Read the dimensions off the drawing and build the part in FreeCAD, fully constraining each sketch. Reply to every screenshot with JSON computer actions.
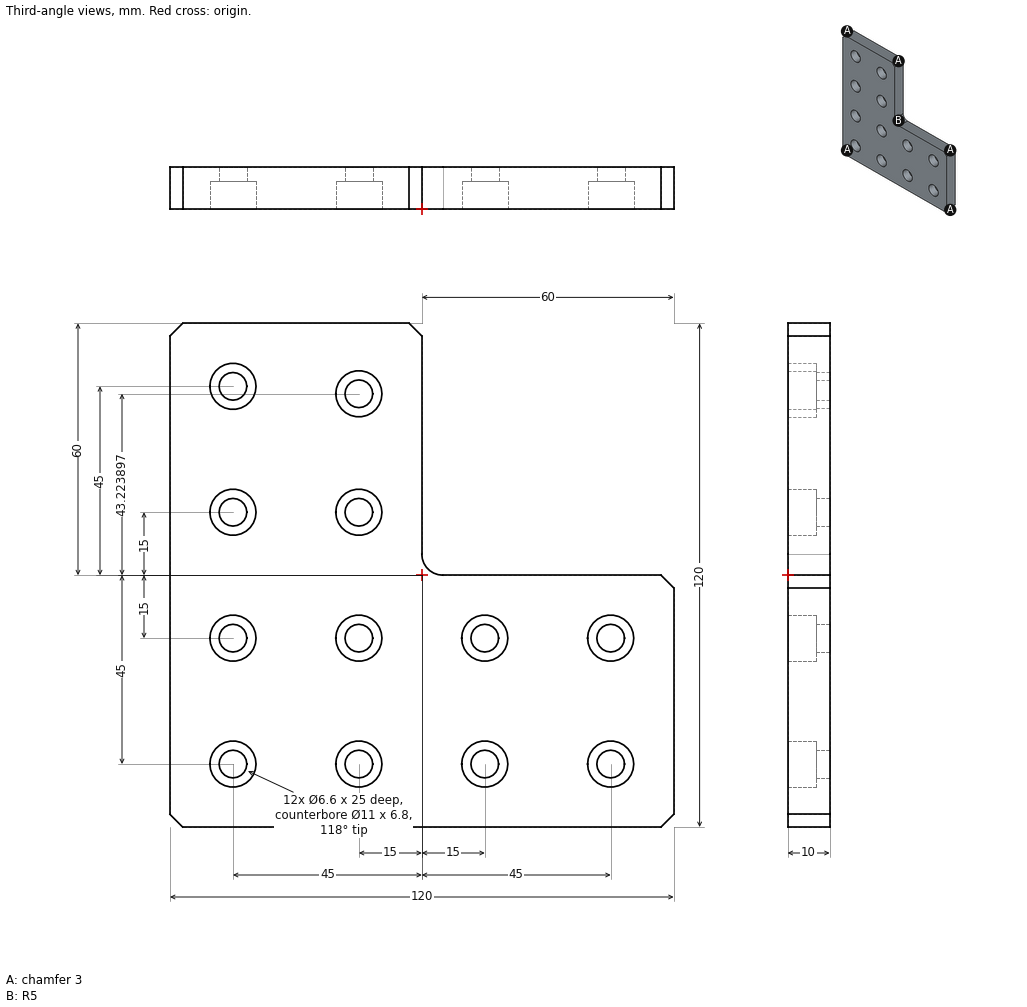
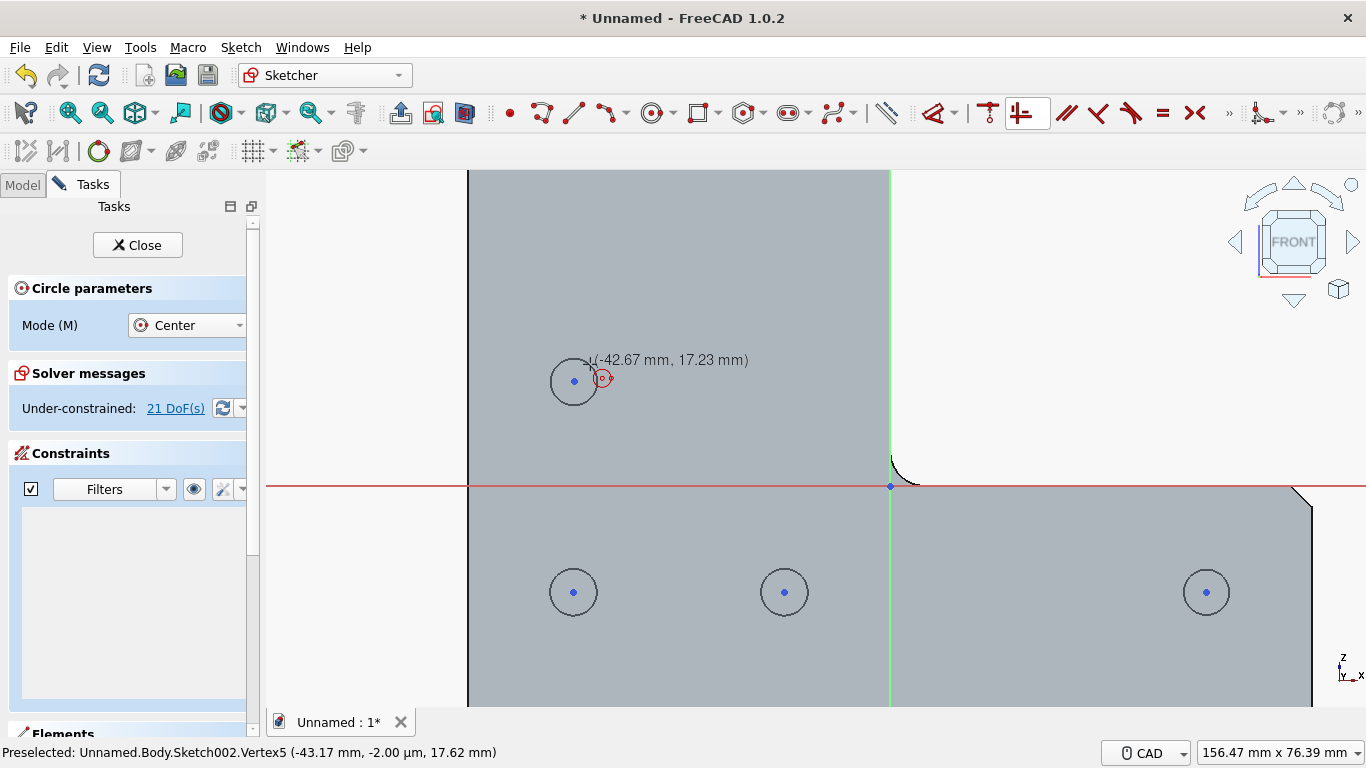
{"action": "scroll", "coordinate": [574, 381], "scroll_direction": "down", "scroll_amount": 3}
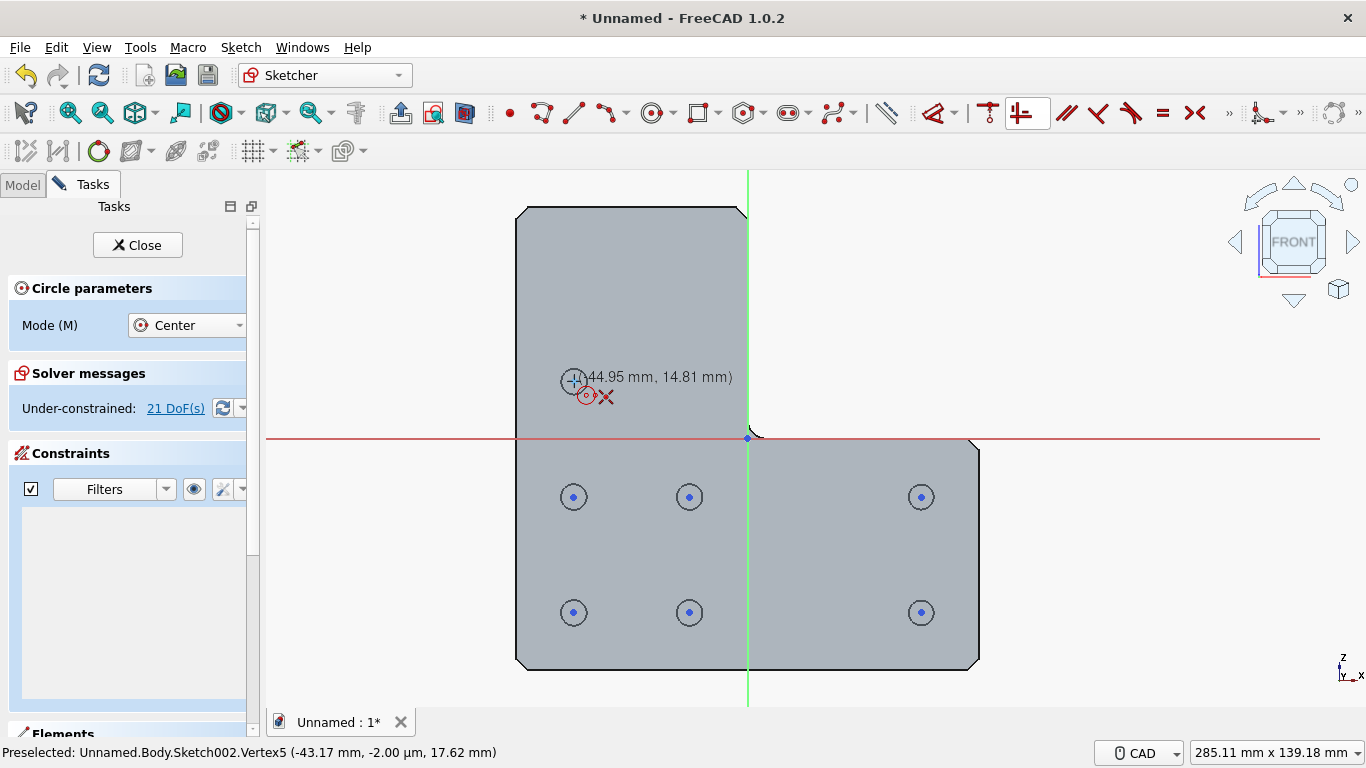
{"action": "scroll", "coordinate": [574, 265], "scroll_direction": "up", "scroll_amount": 3}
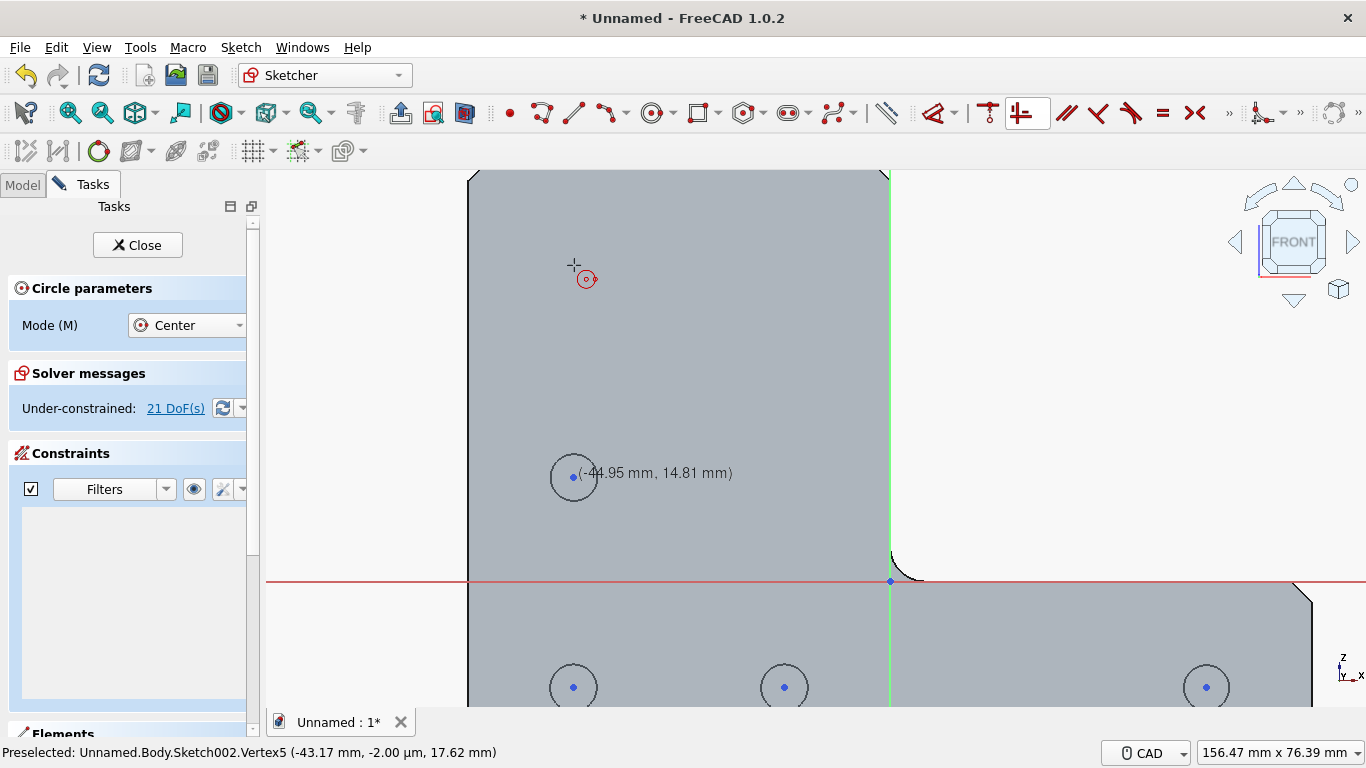
{"action": "left_click", "coordinate": [574, 265]}
{"action": "left_click", "coordinate": [590, 249]}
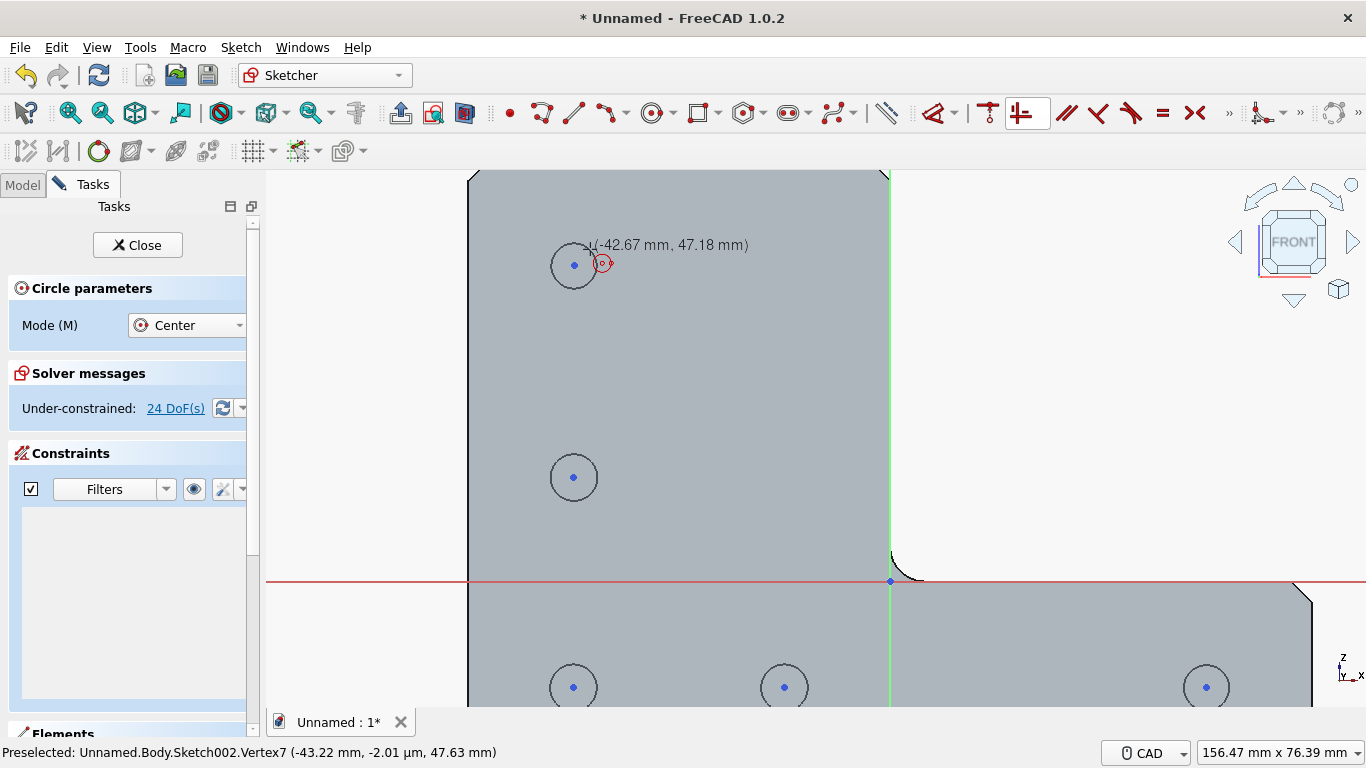
{"action": "left_click", "coordinate": [785, 278]}
{"action": "left_click", "coordinate": [801, 261]}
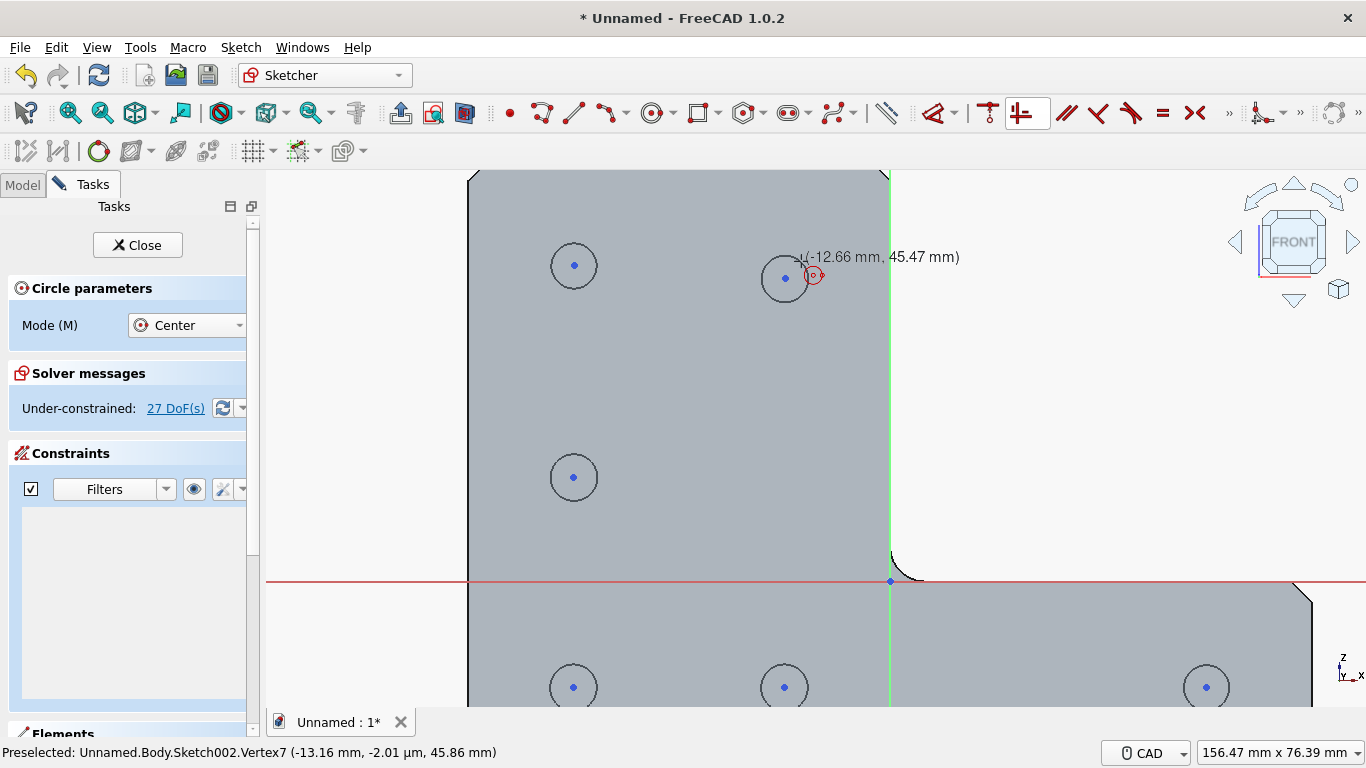
{"action": "left_click", "coordinate": [785, 476]}
{"action": "left_click", "coordinate": [801, 460]}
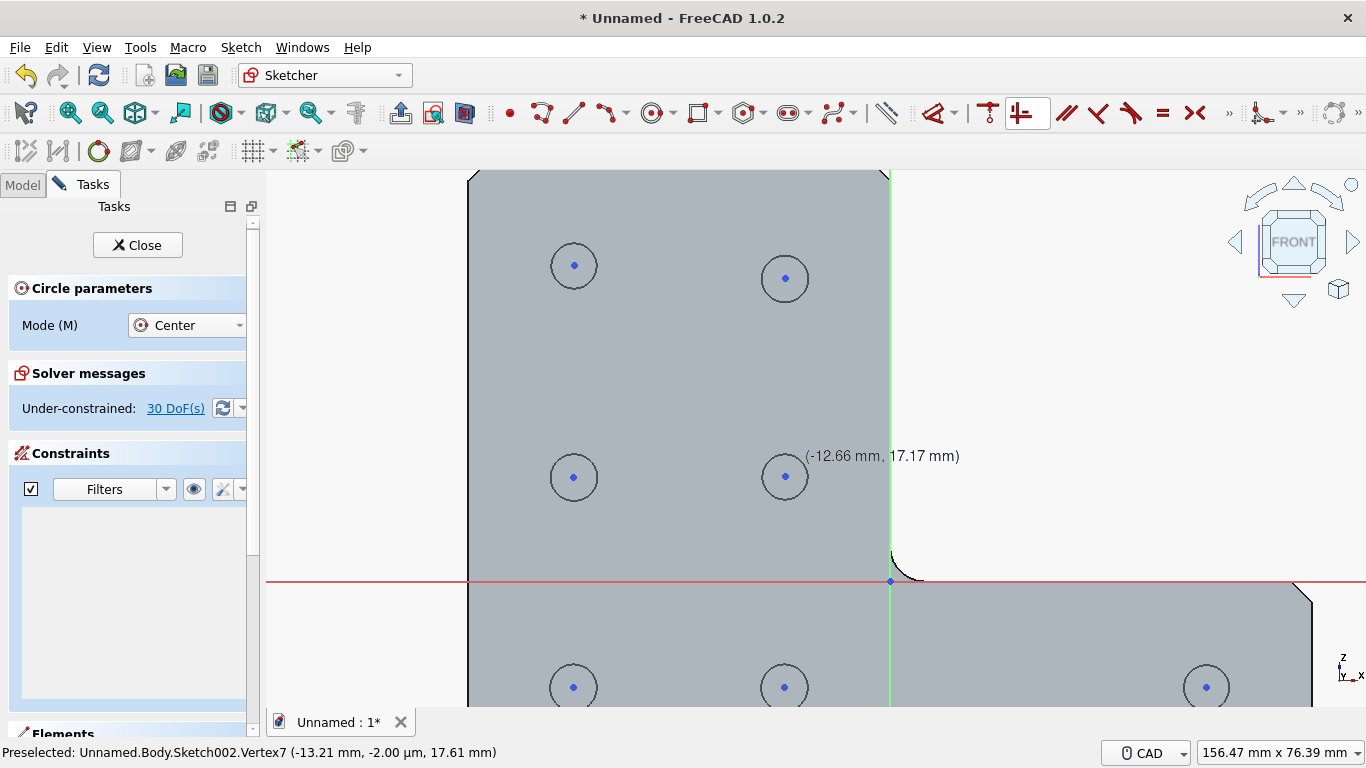
{"action": "scroll", "coordinate": [574, 264], "scroll_direction": "down", "scroll_amount": 3}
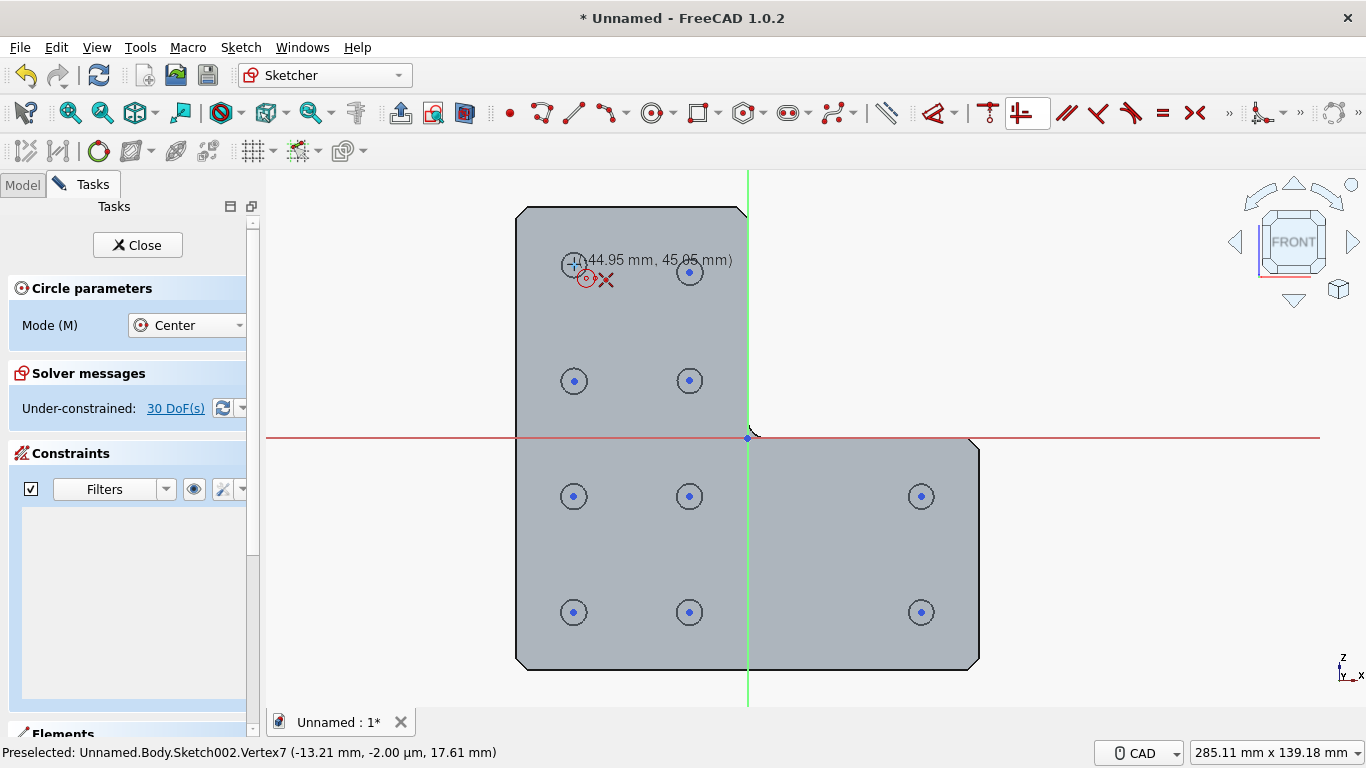
{"action": "scroll", "coordinate": [805, 612], "scroll_direction": "up", "scroll_amount": 3}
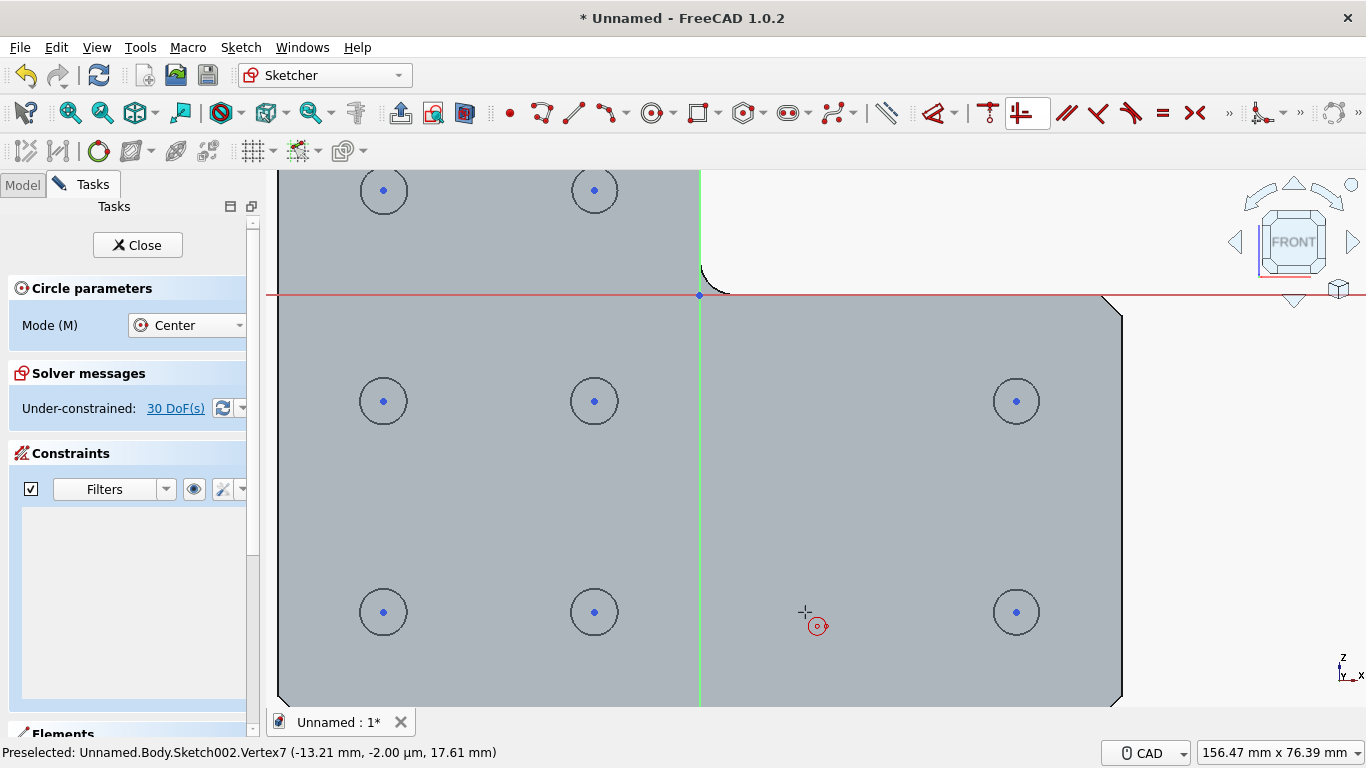
{"action": "left_click", "coordinate": [805, 611]}
{"action": "left_click", "coordinate": [822, 595]}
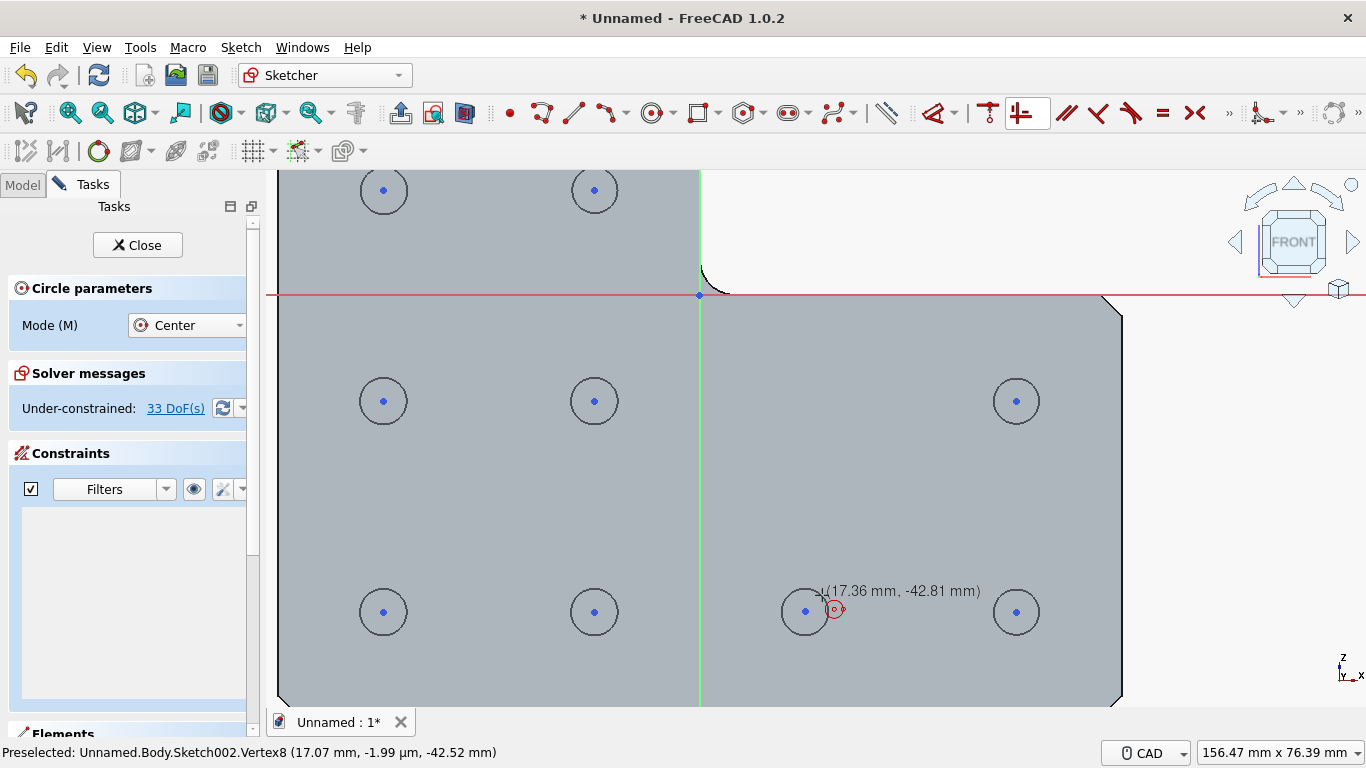
{"action": "left_click", "coordinate": [805, 400]}
{"action": "left_click", "coordinate": [822, 384]}
{"action": "key", "text": "Escape"}